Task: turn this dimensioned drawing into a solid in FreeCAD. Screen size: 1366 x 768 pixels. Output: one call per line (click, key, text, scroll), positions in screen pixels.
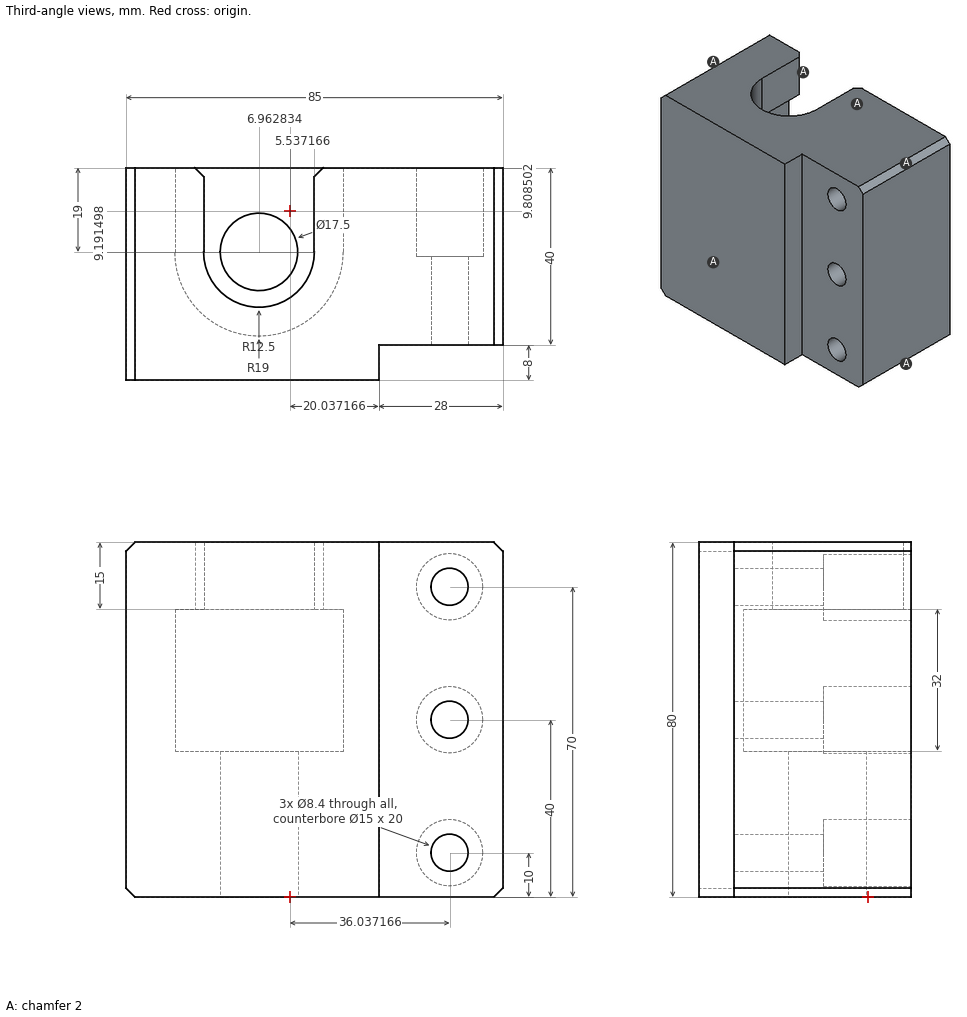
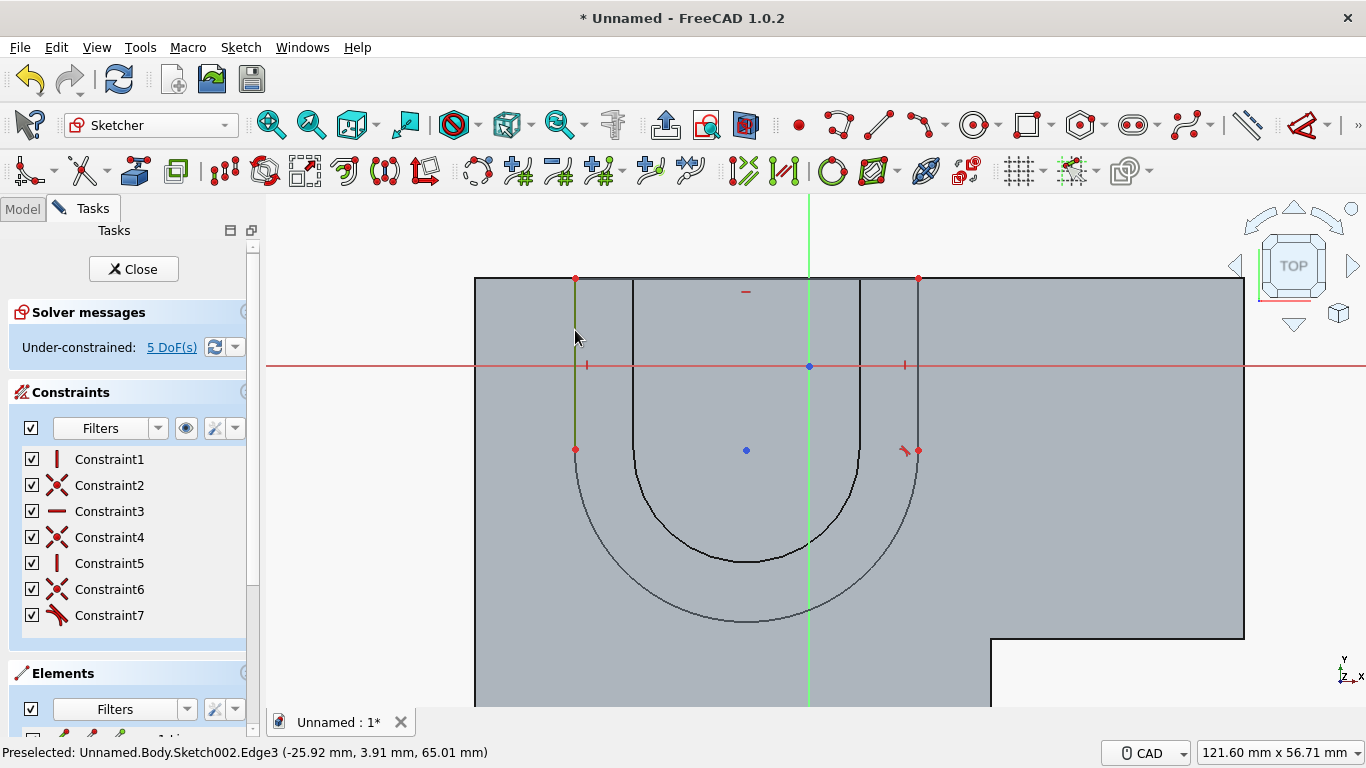
click(645, 589)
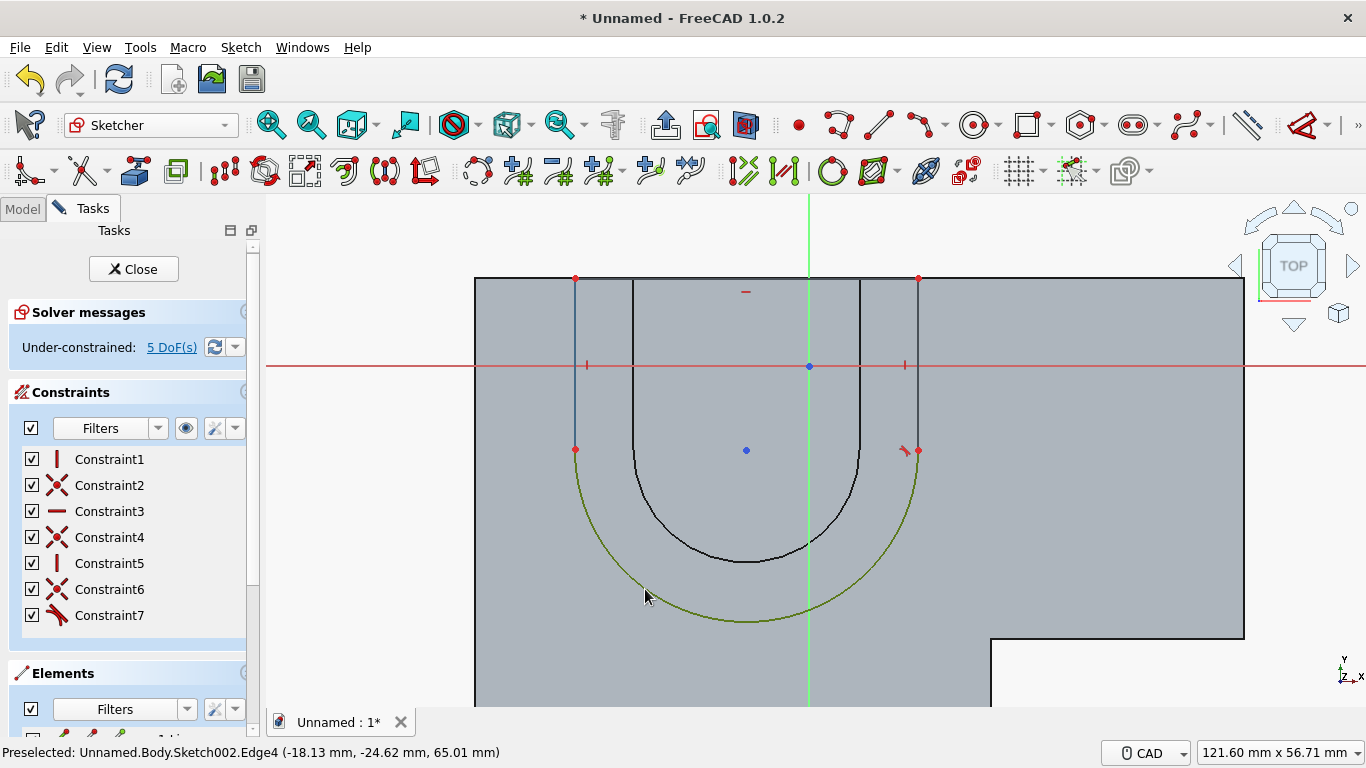
key(t)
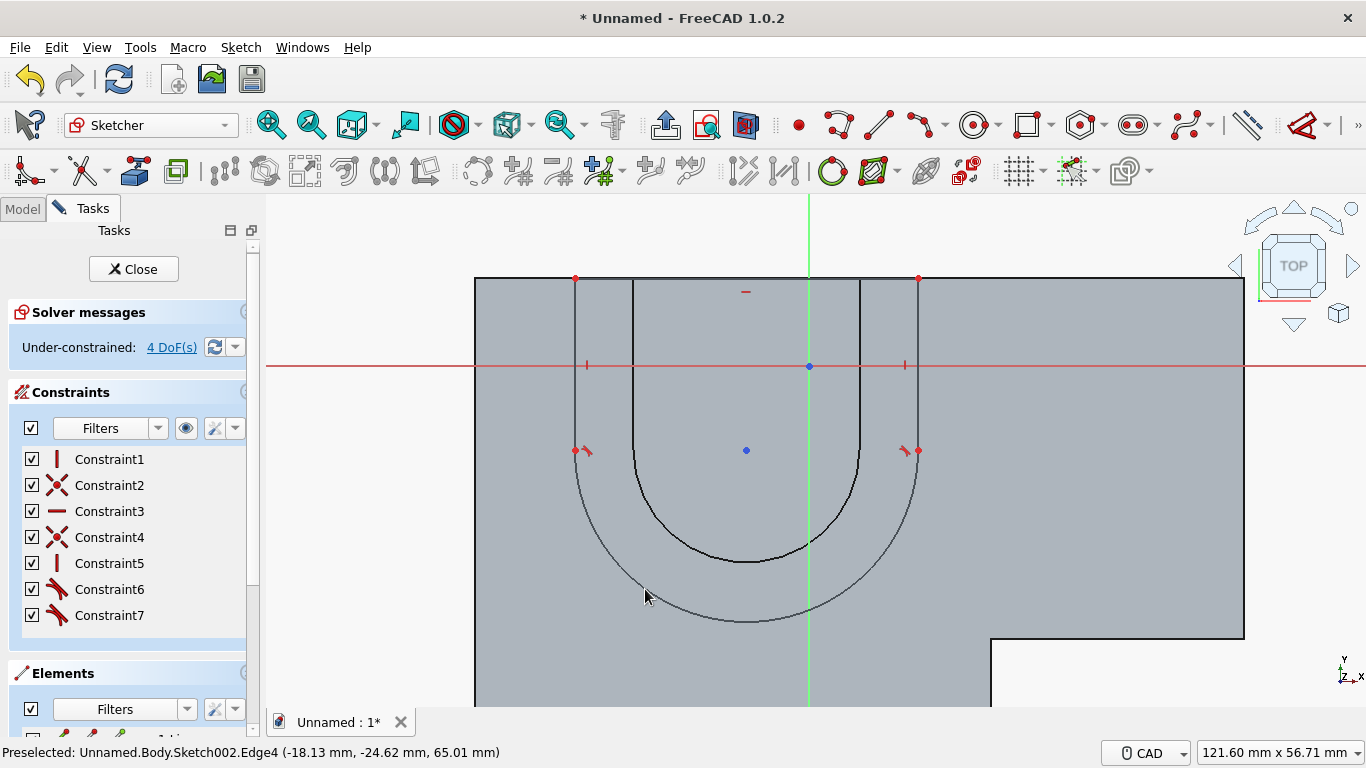
click(1302, 126)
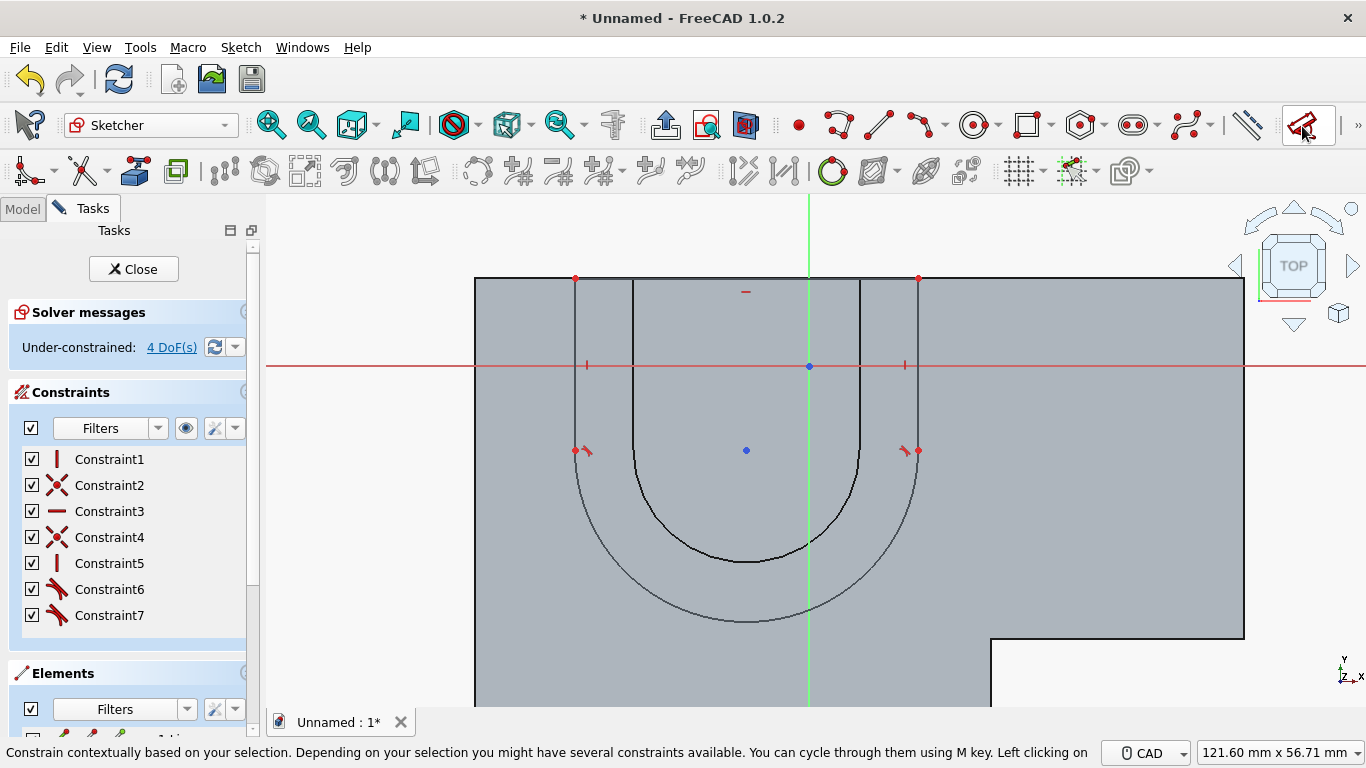
click(646, 589)
click(627, 615)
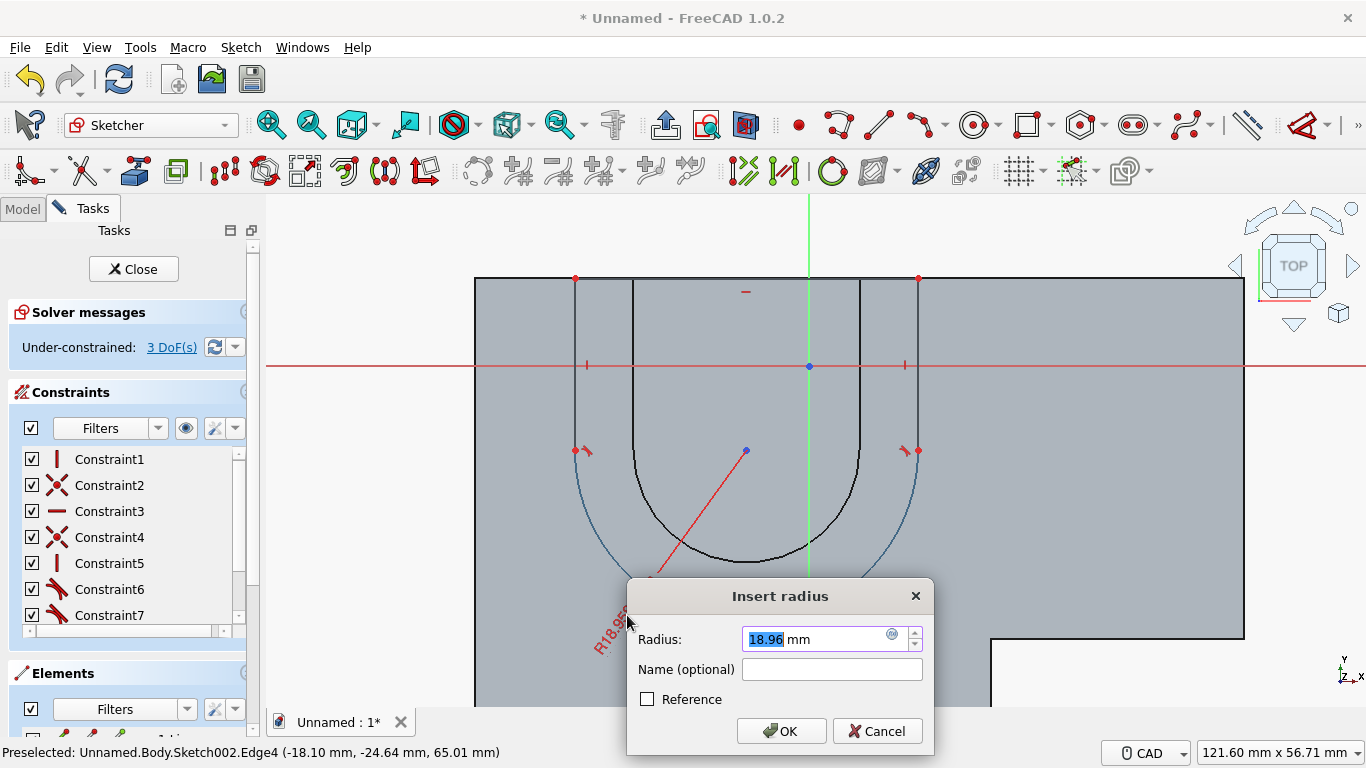
text(19)
key(Return)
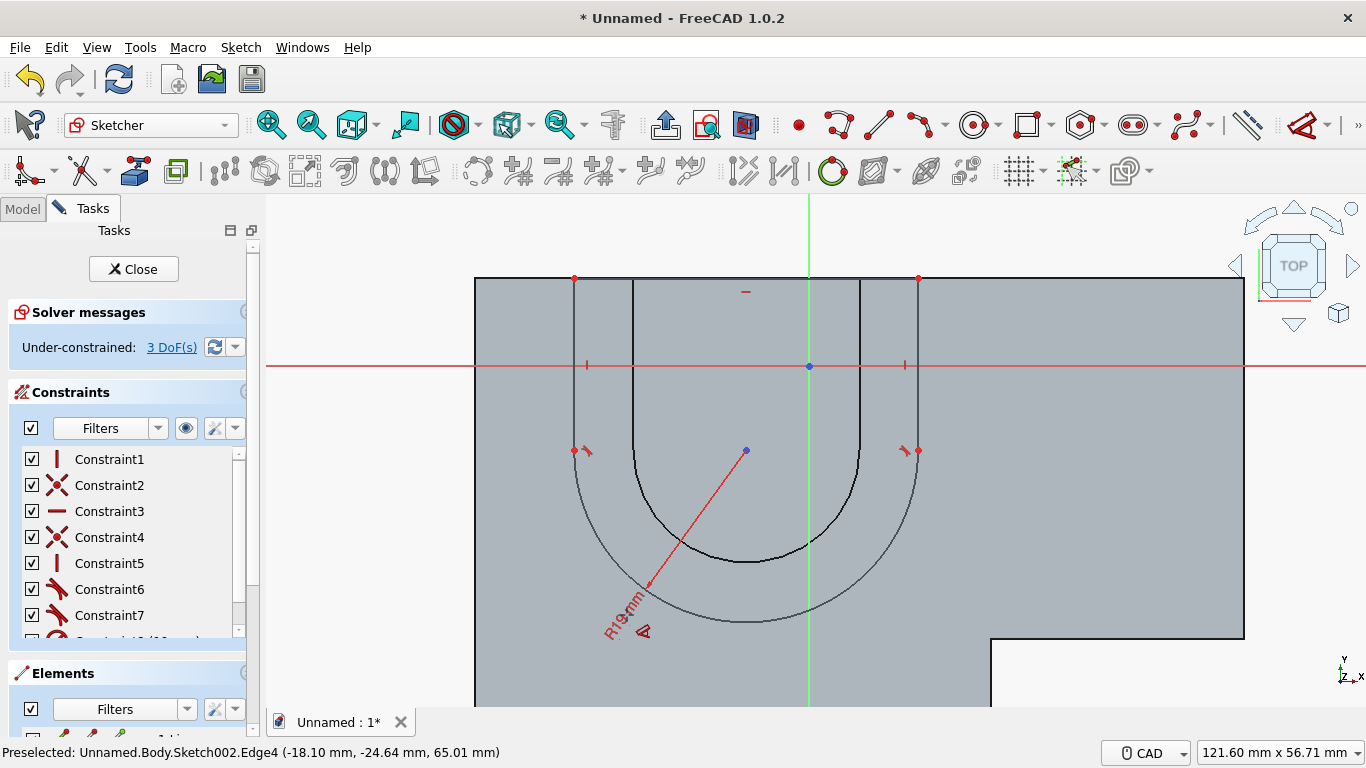
click(918, 399)
click(952, 325)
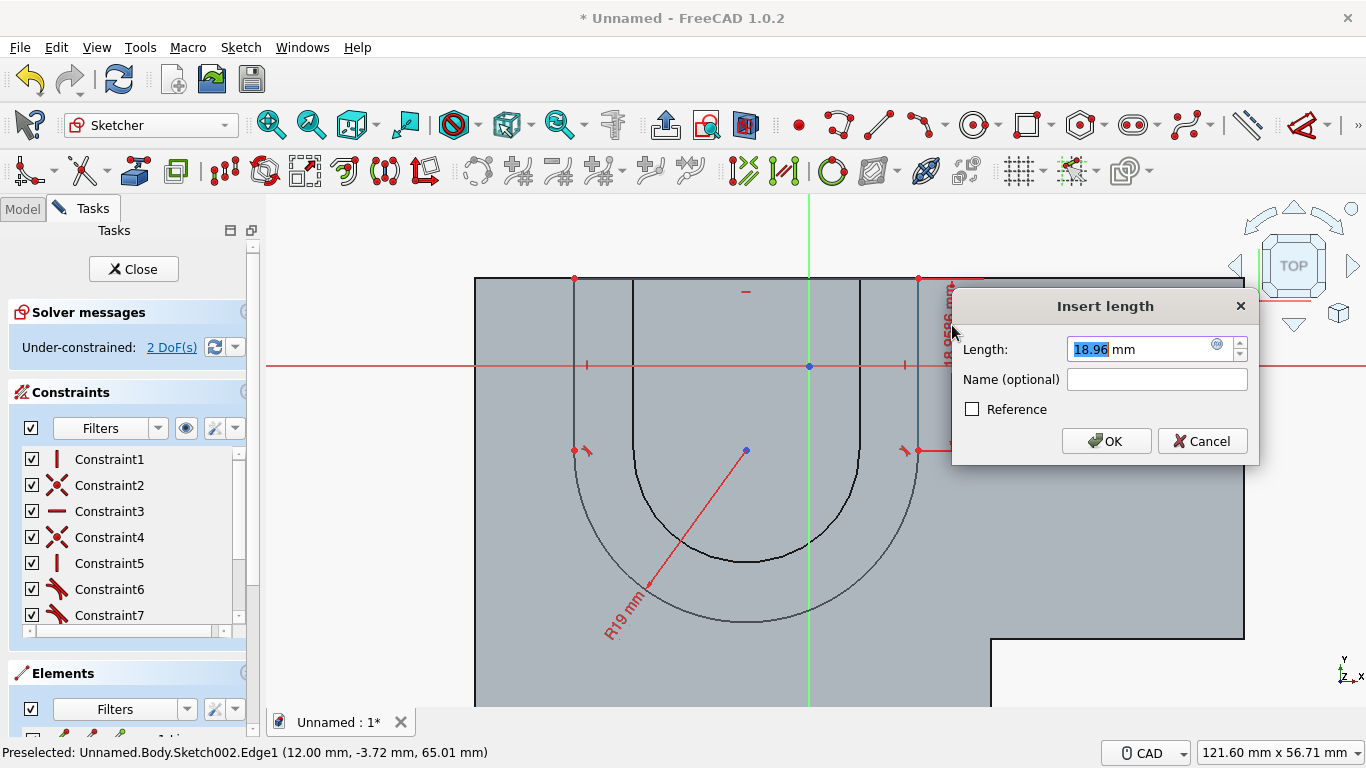
text(19)
key(Return)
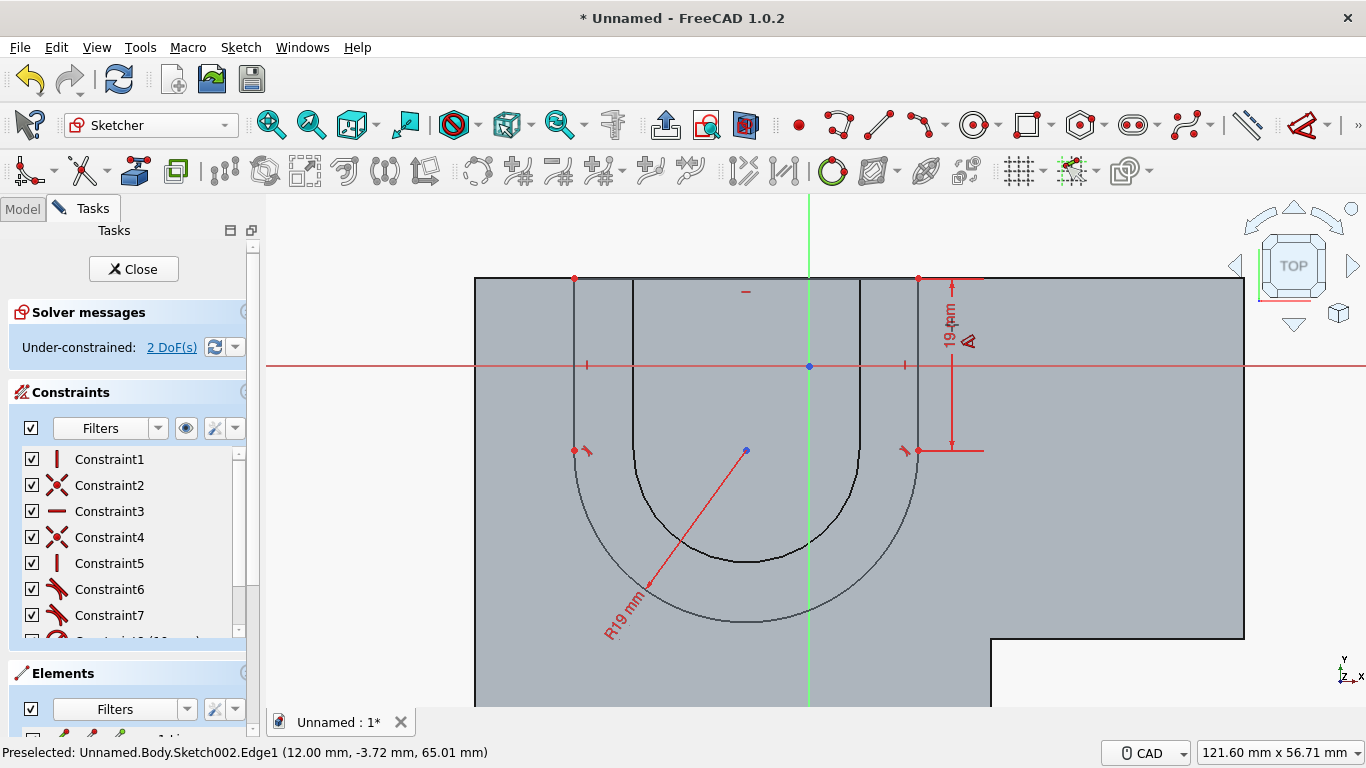
click(918, 451)
click(952, 408)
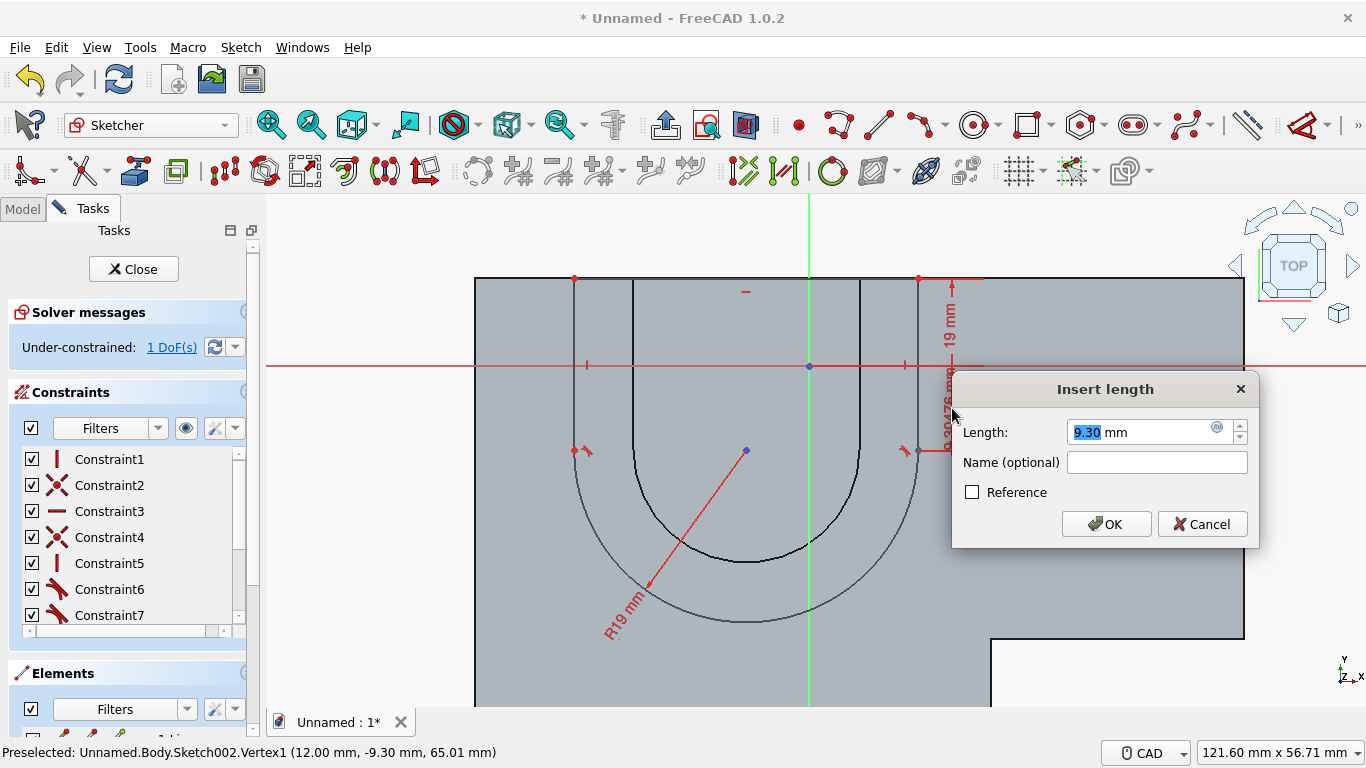
text(9.191498)
key(Return)